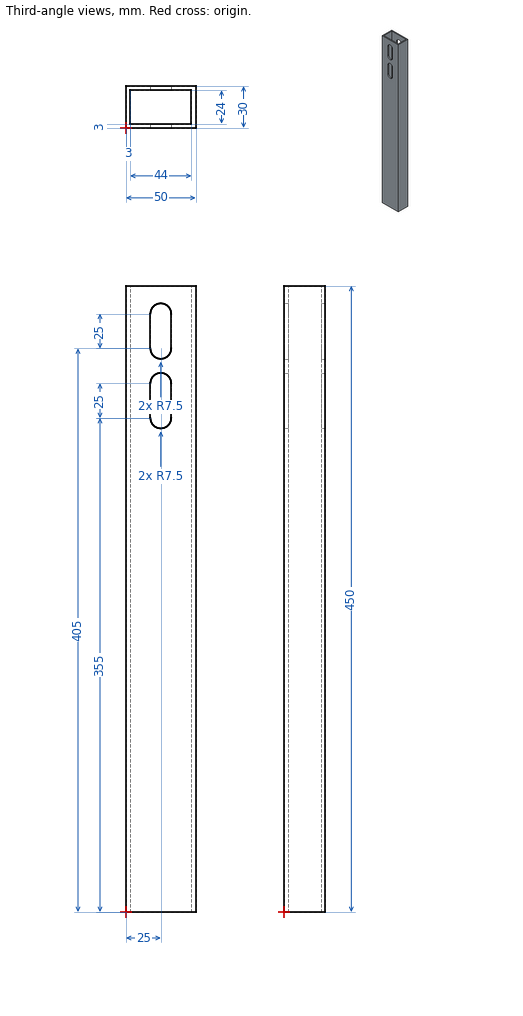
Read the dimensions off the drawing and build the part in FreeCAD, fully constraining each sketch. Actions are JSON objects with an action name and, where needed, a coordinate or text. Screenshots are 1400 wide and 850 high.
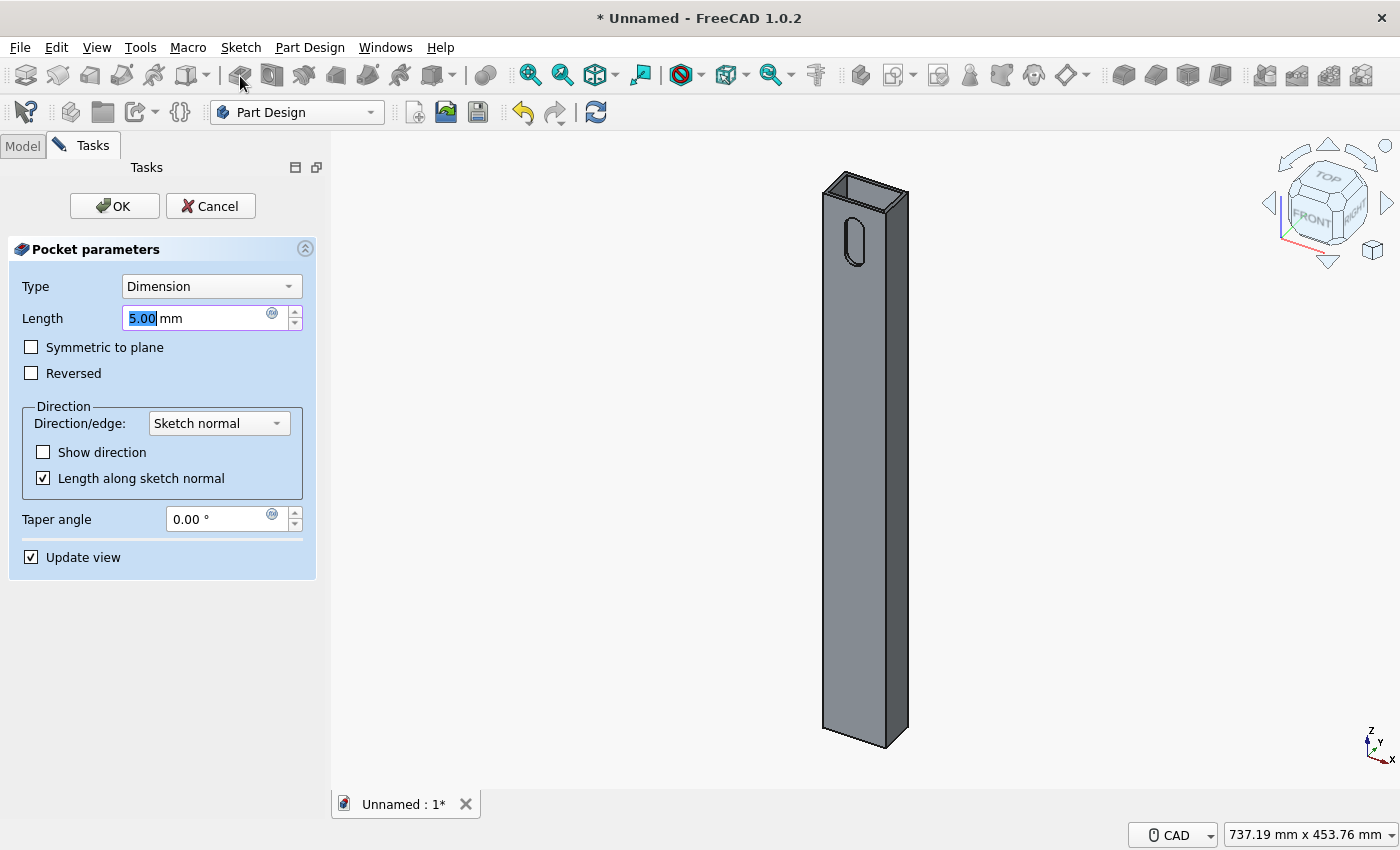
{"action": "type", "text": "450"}
{"action": "key", "text": "Tab"}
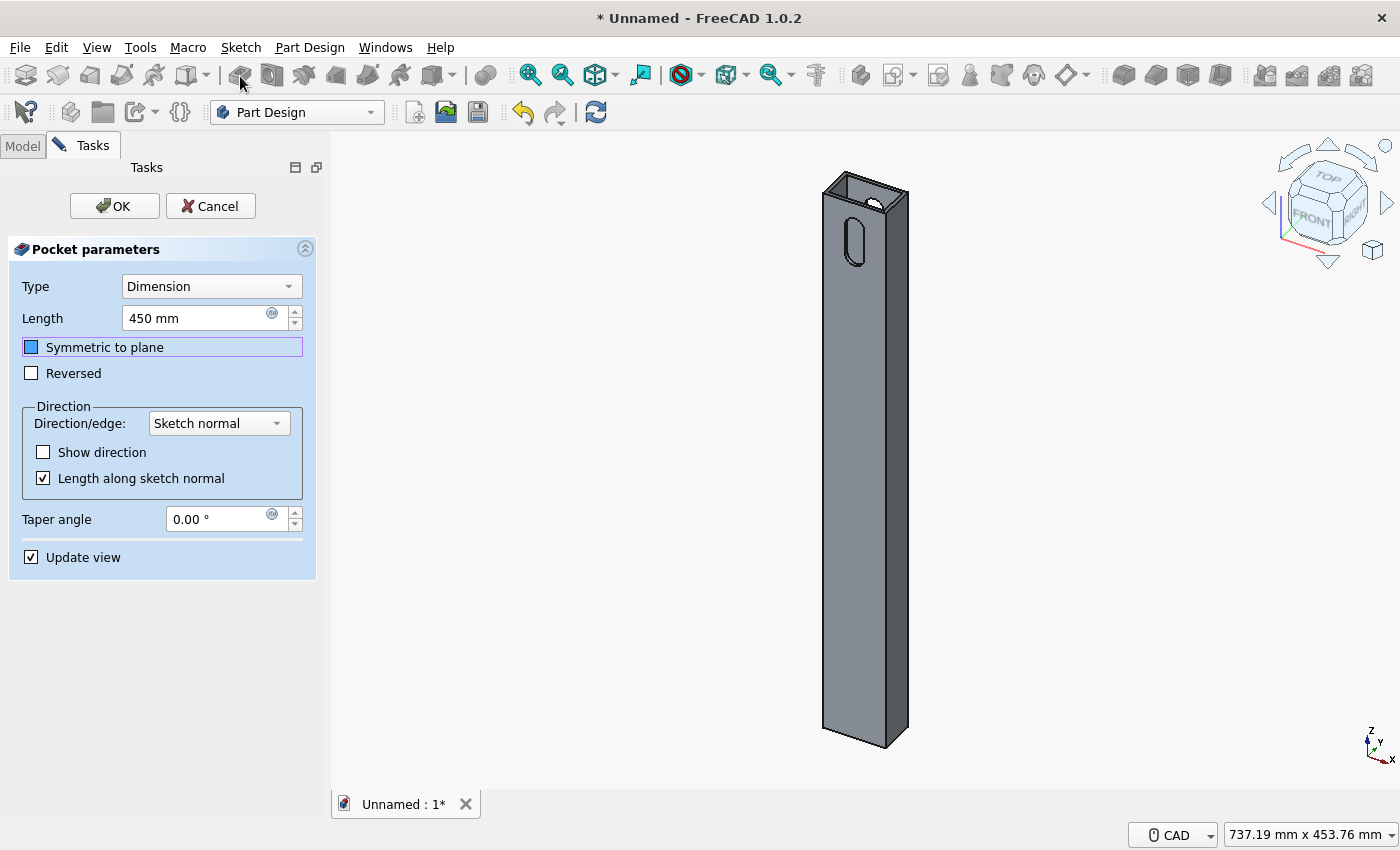
{"action": "left_click", "coordinate": [115, 206]}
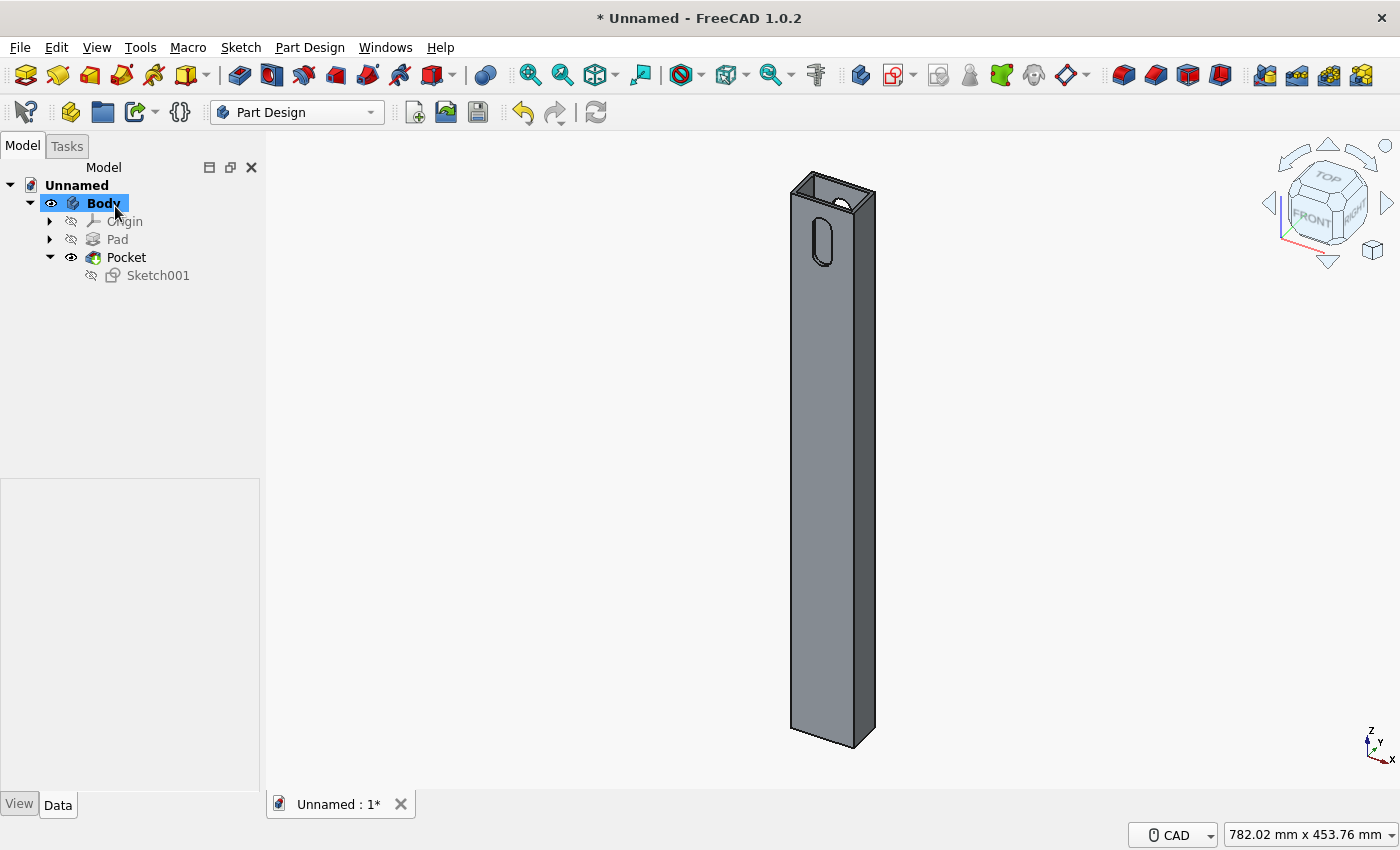
{"action": "left_click", "coordinate": [894, 76]}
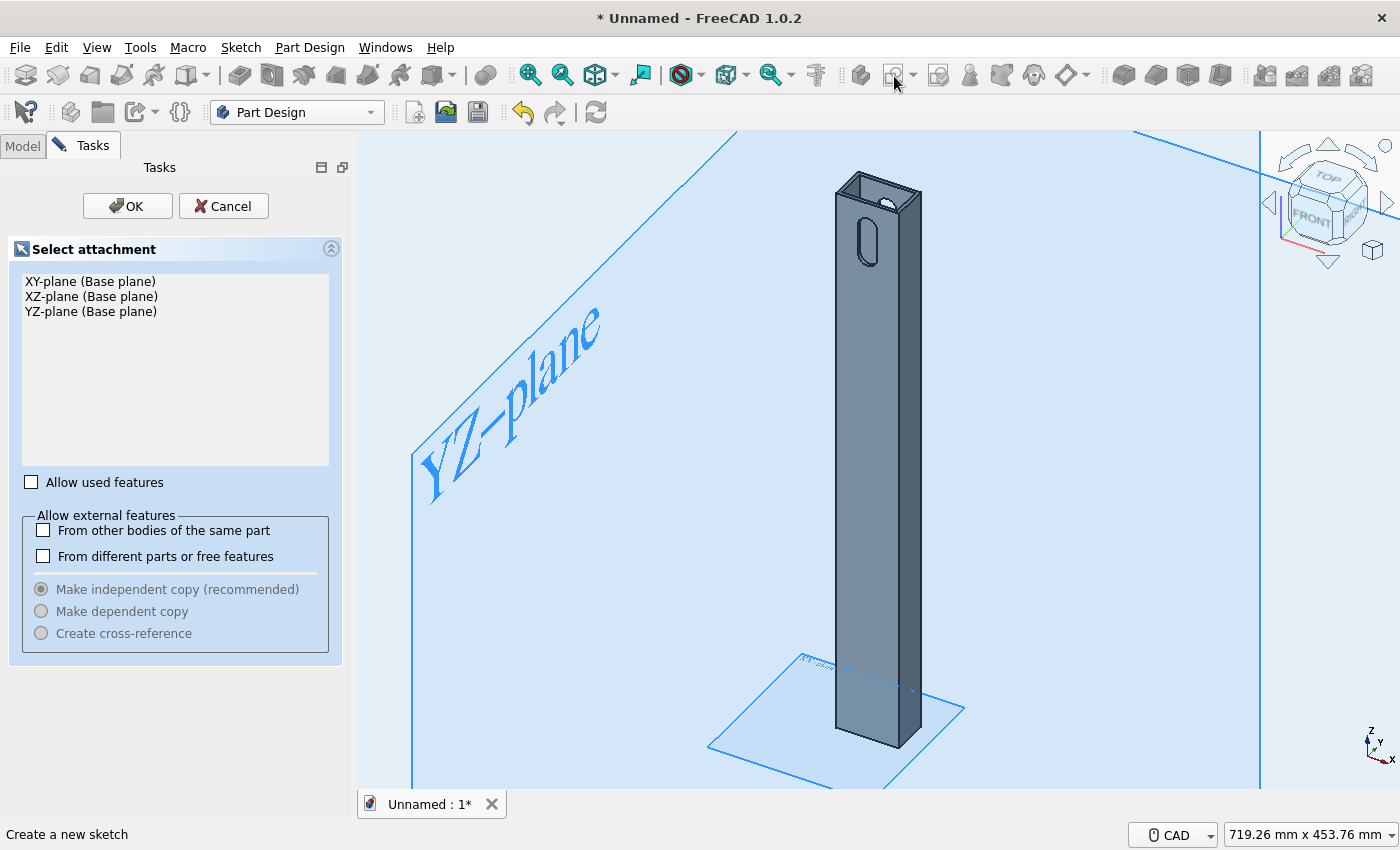
{"action": "left_click", "coordinate": [82, 296]}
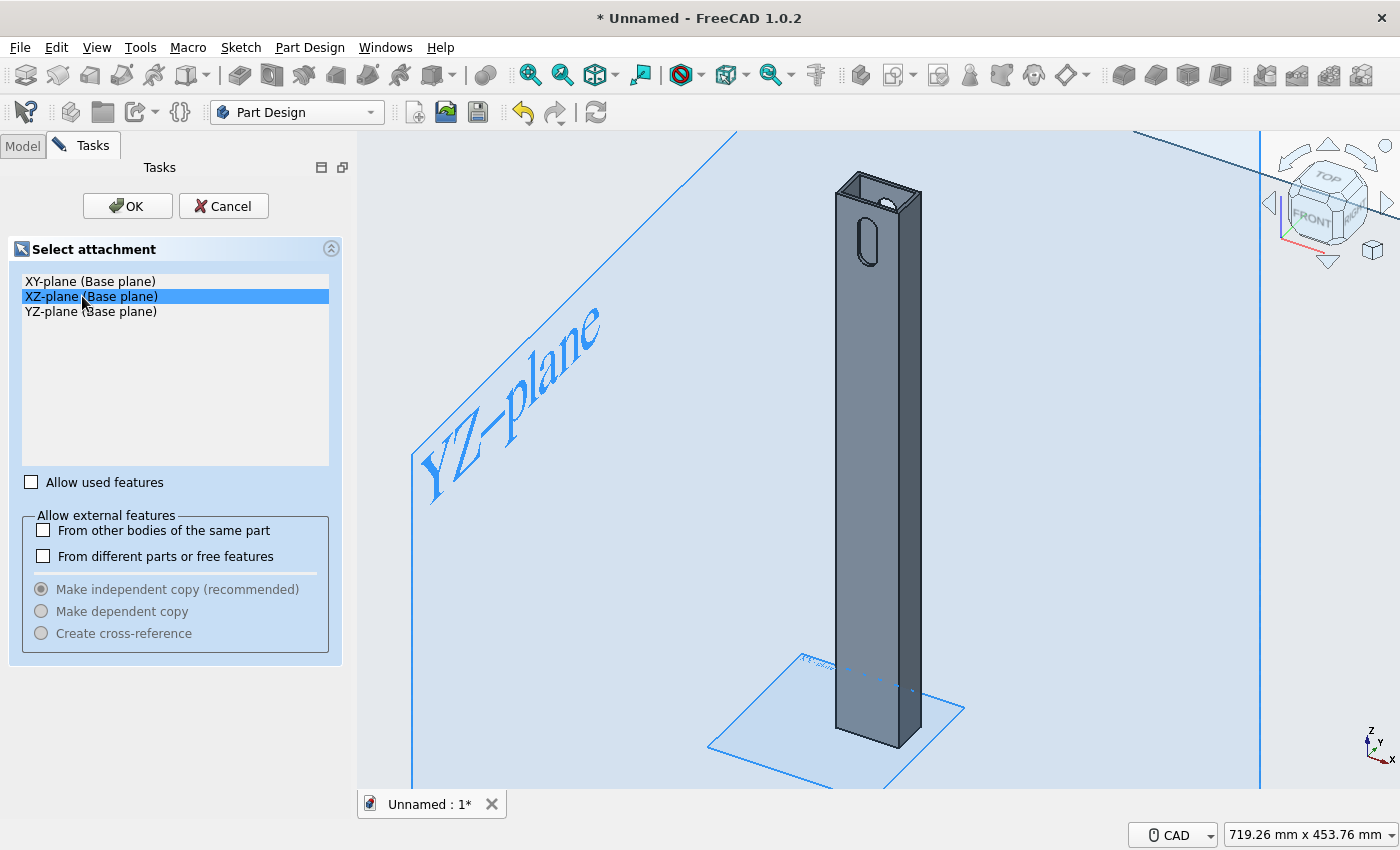
{"action": "left_click", "coordinate": [128, 206]}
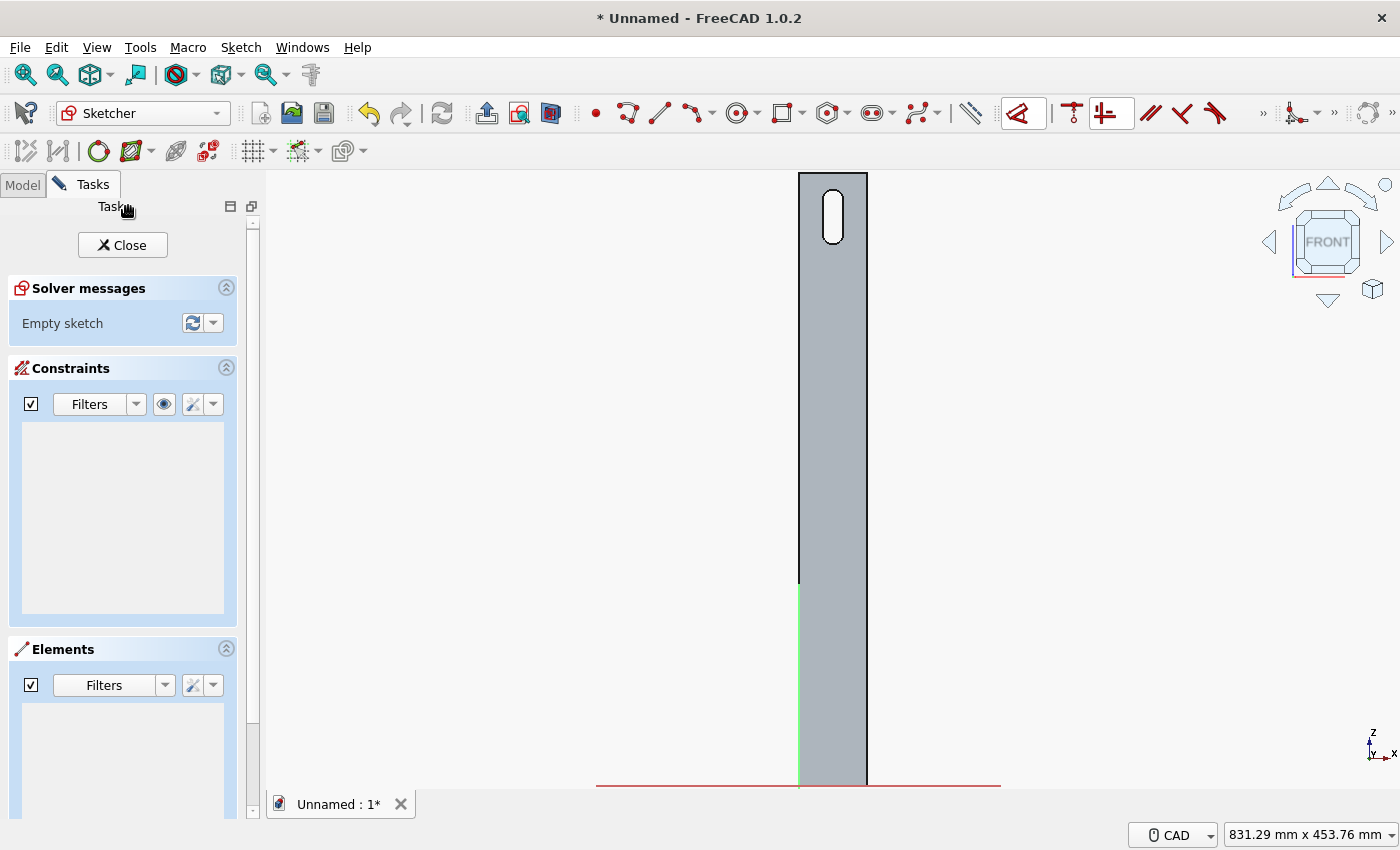
{"action": "scroll", "coordinate": [844, 255], "scroll_direction": "up", "scroll_amount": 10}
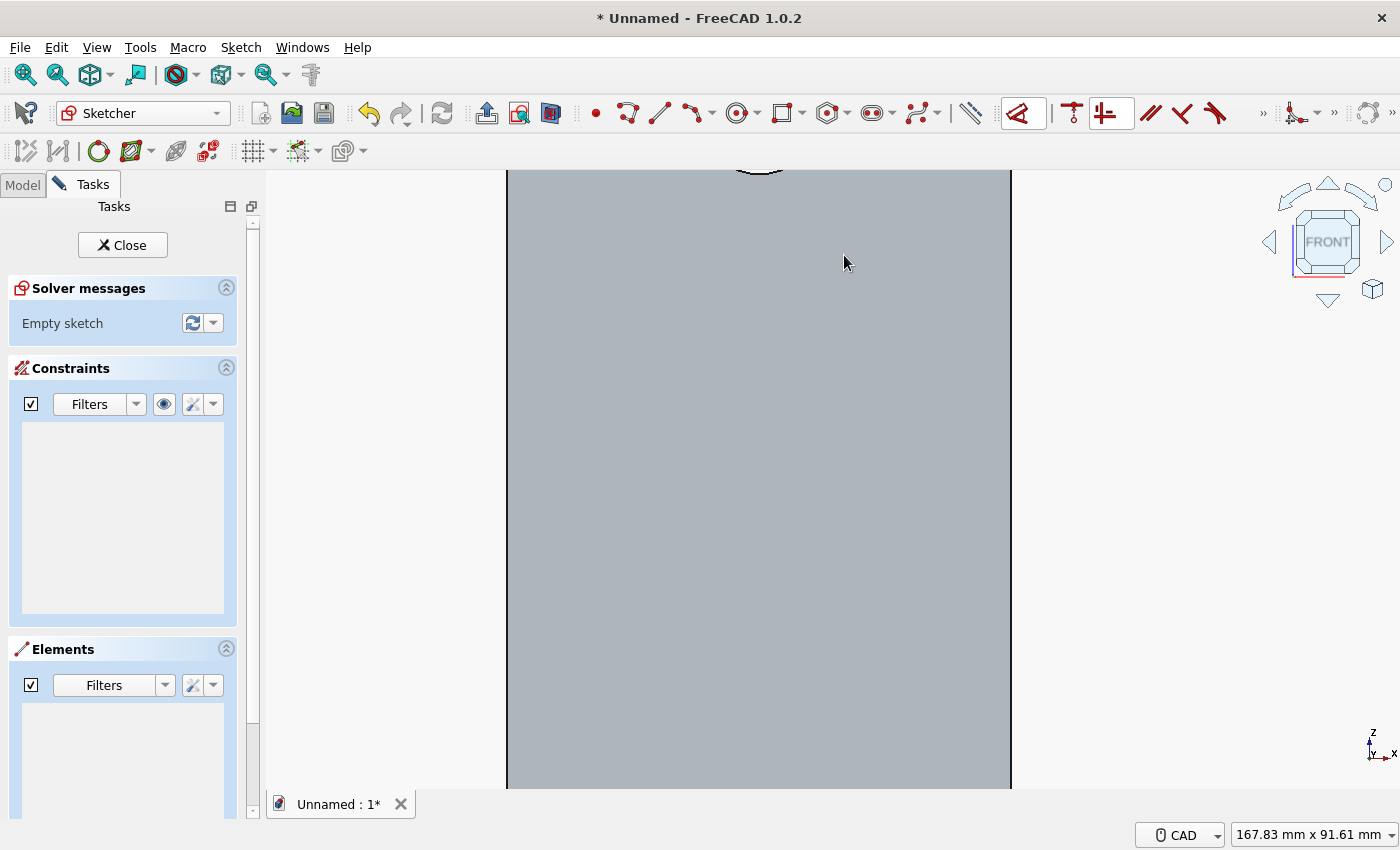
{"action": "key", "text": "g s"}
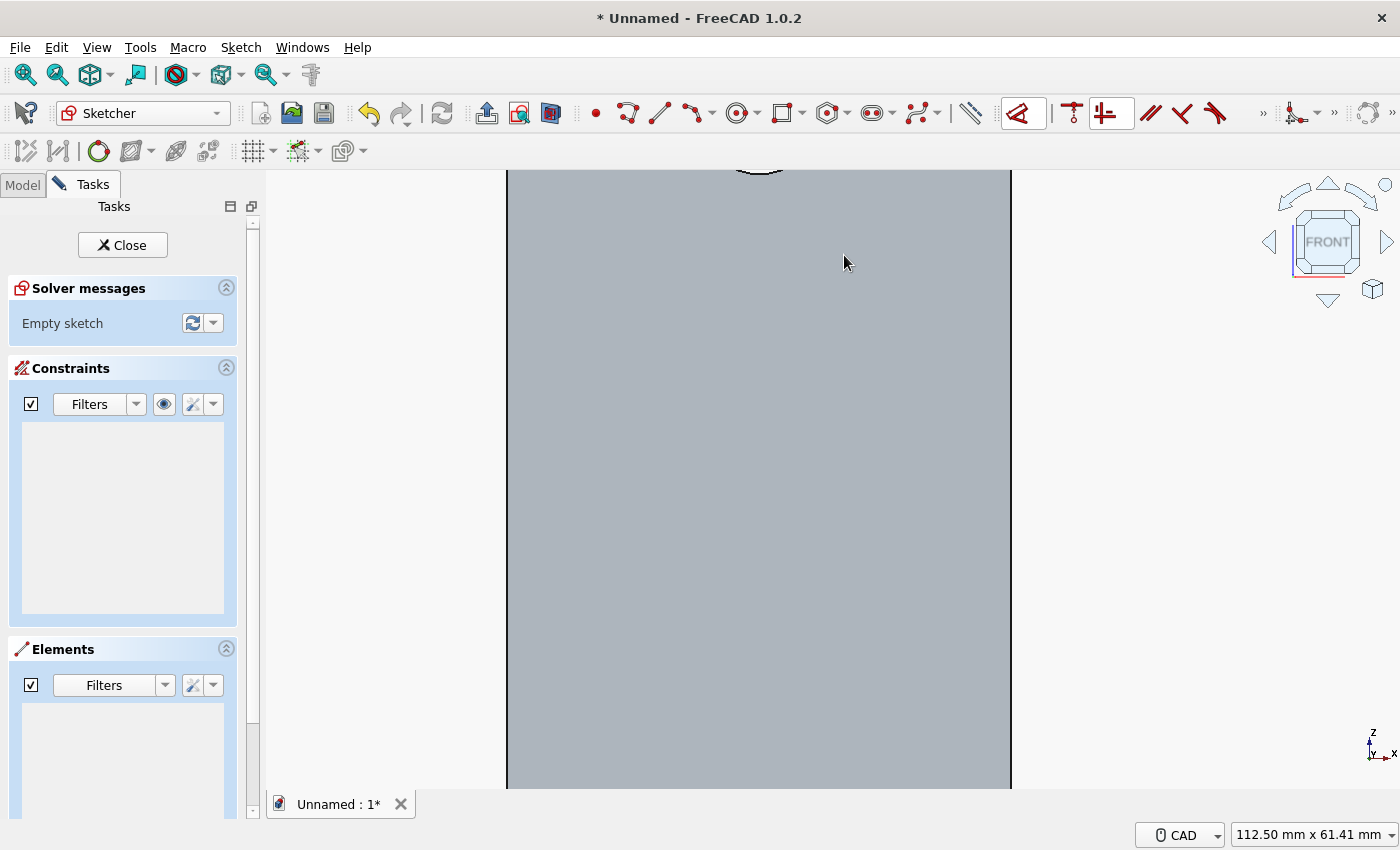
{"action": "left_click", "coordinate": [759, 603]}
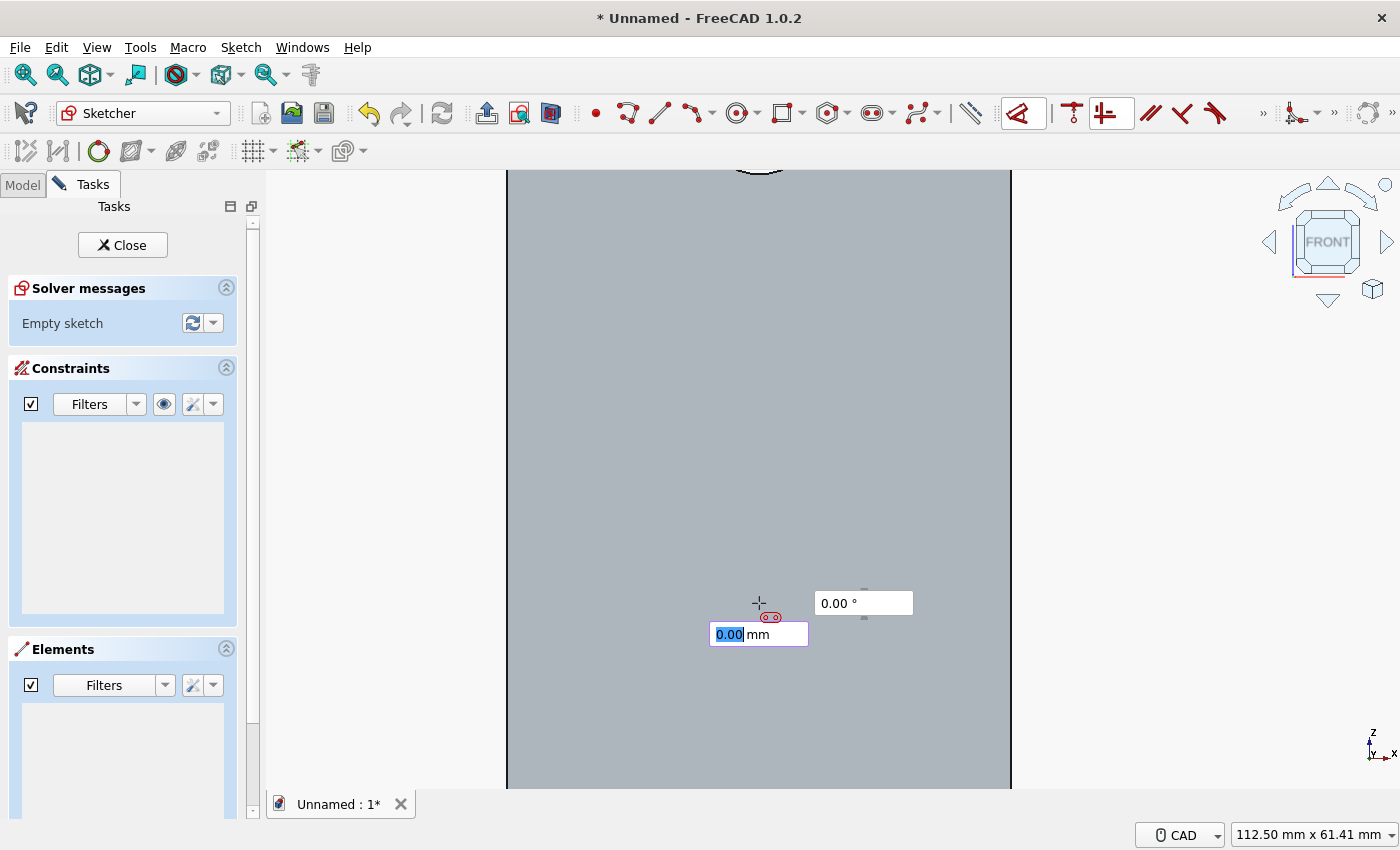
{"action": "left_click", "coordinate": [759, 351]}